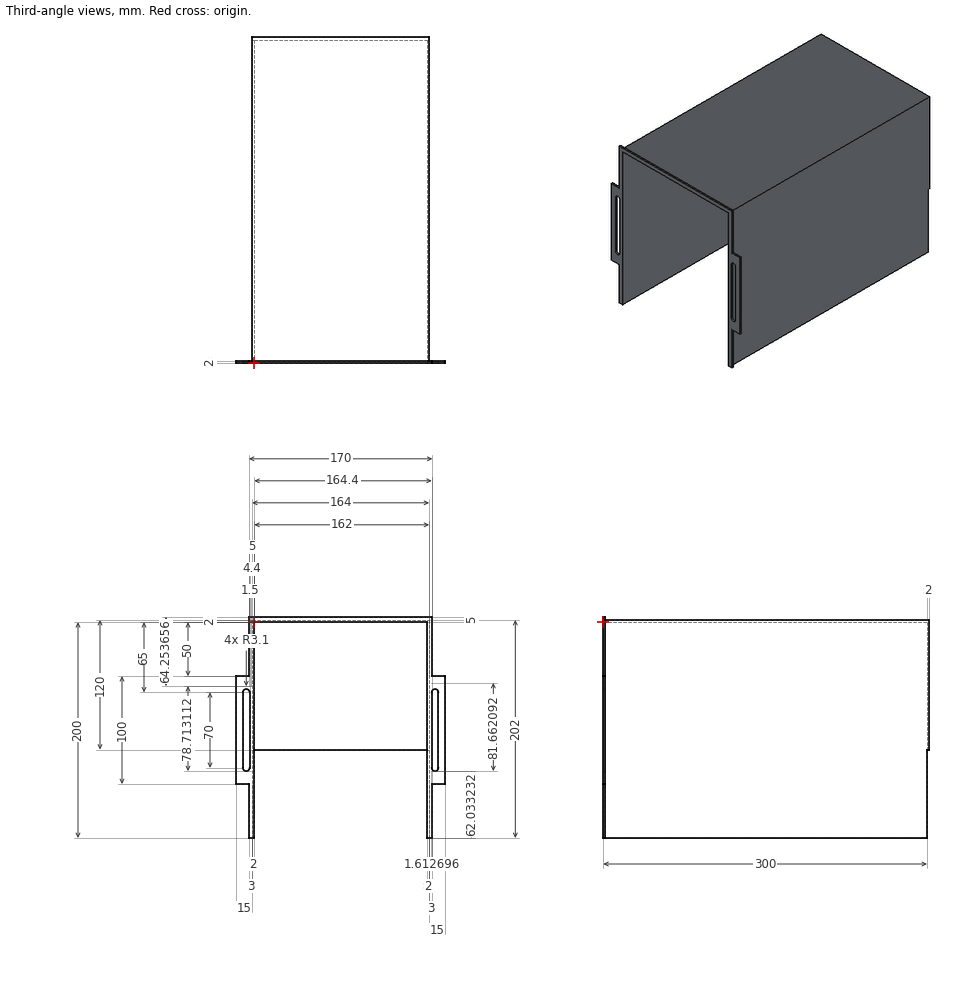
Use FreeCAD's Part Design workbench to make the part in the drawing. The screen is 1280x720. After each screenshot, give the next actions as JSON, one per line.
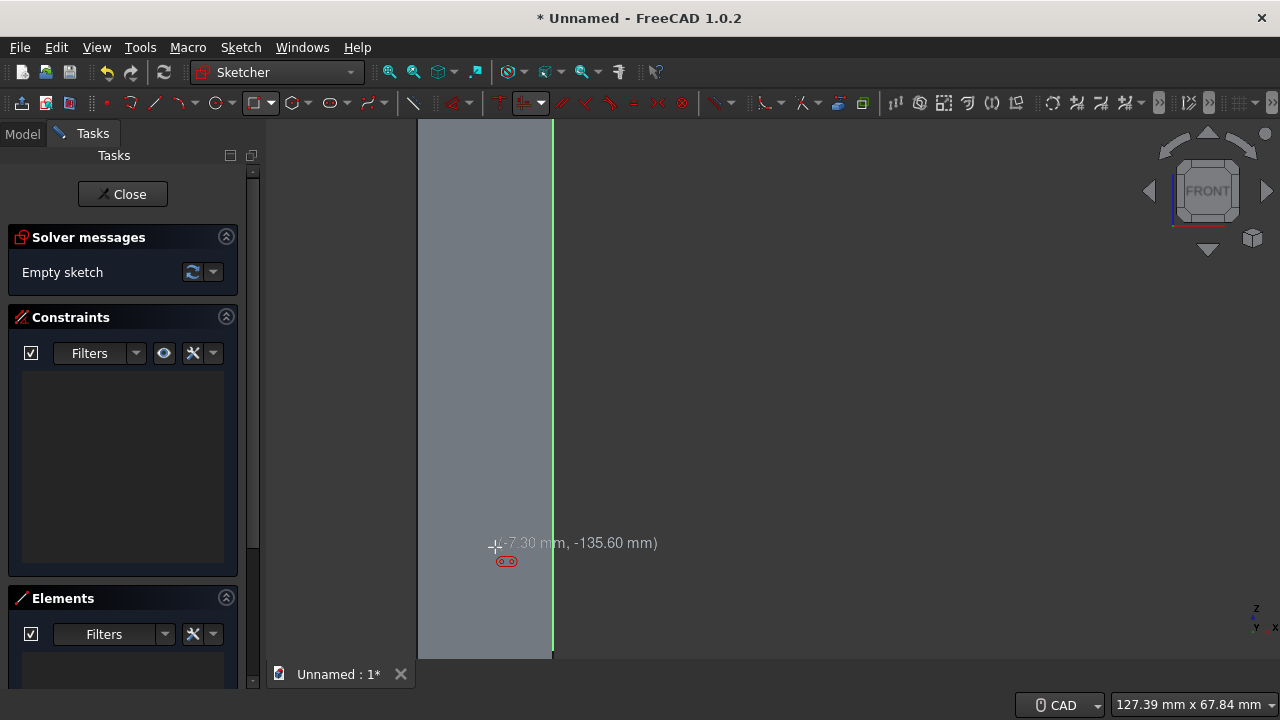
{"action": "left_click", "coordinate": [493, 544]}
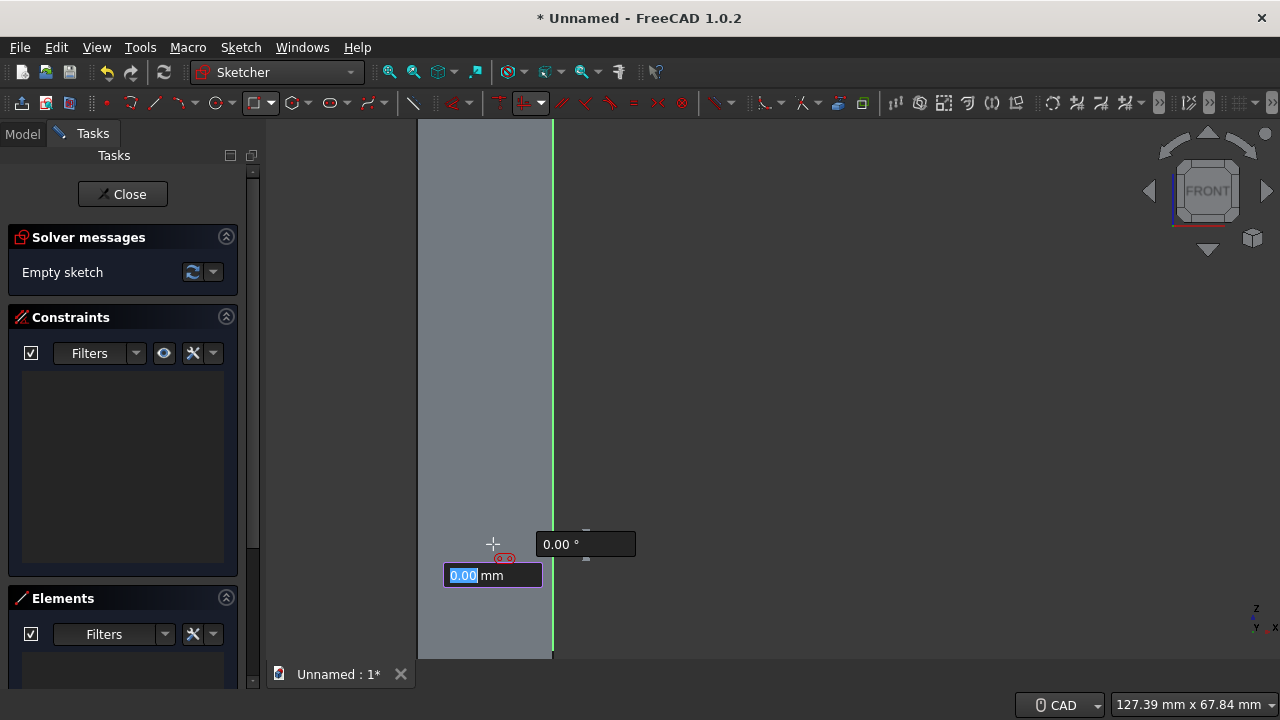
{"action": "scroll", "coordinate": [496, 549], "scroll_direction": "down", "scroll_amount": 6}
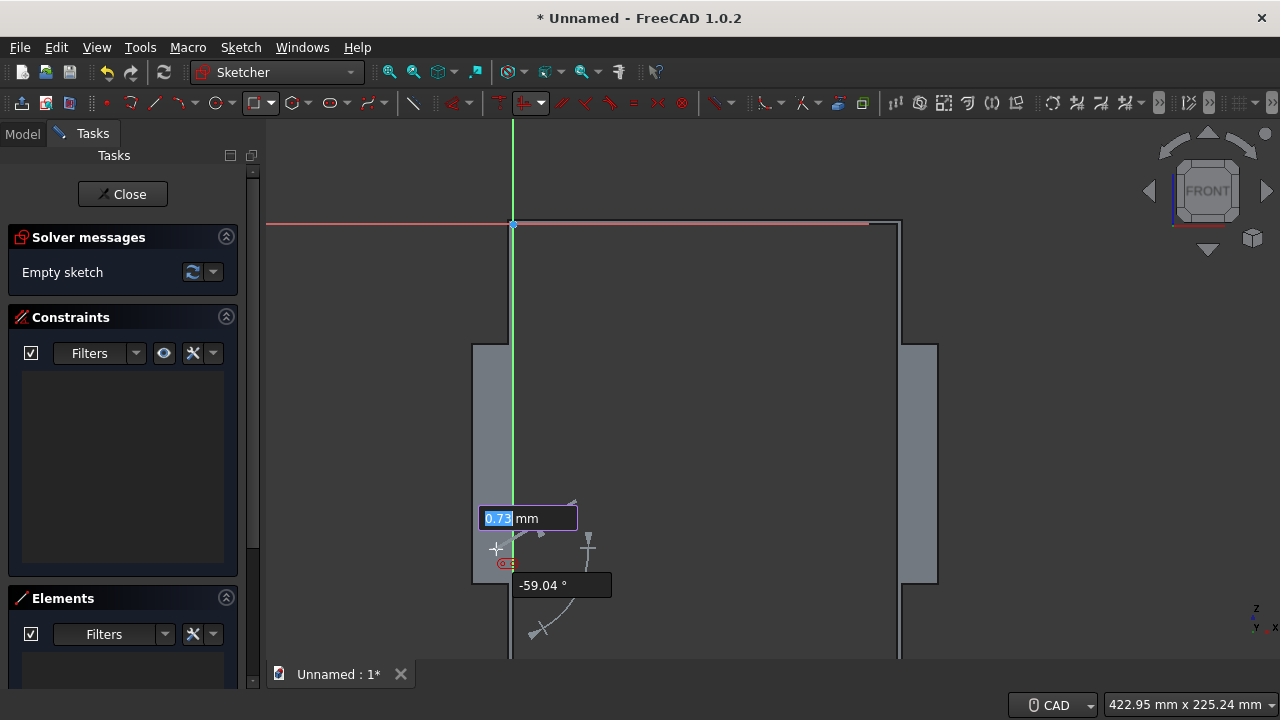
{"action": "left_click", "coordinate": [495, 380]}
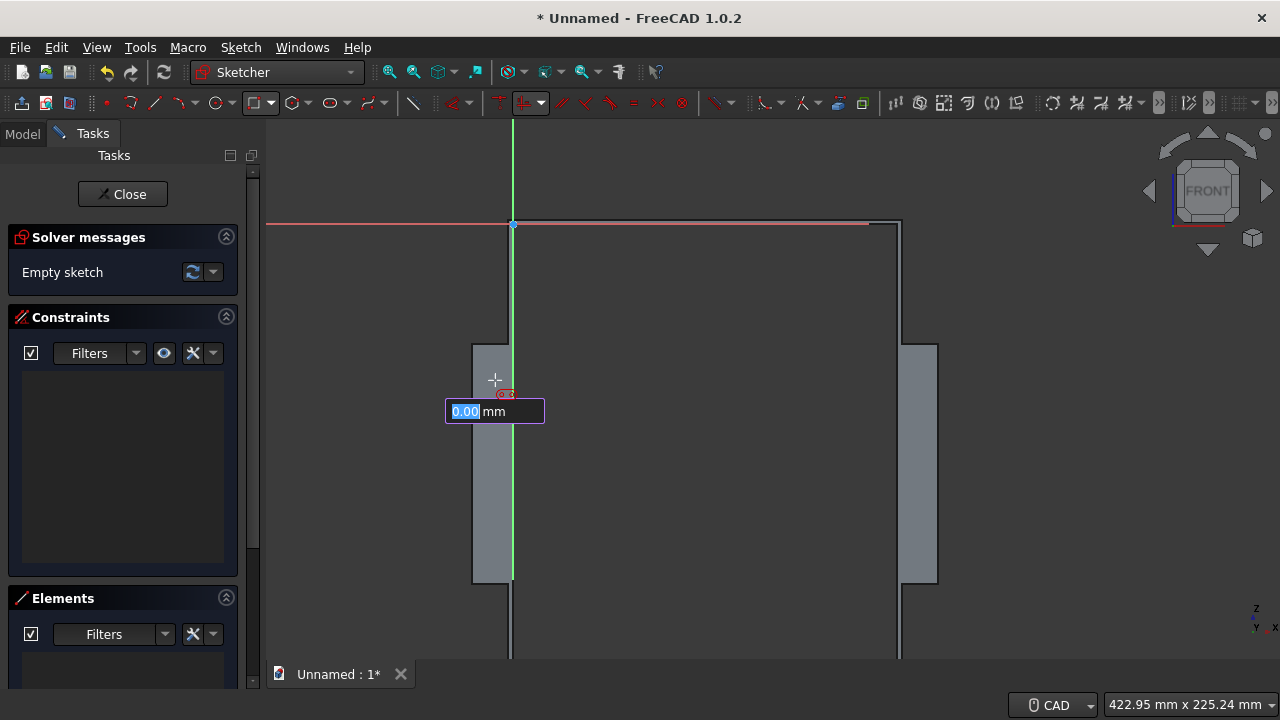
{"action": "scroll", "coordinate": [488, 464], "scroll_direction": "up", "scroll_amount": 4}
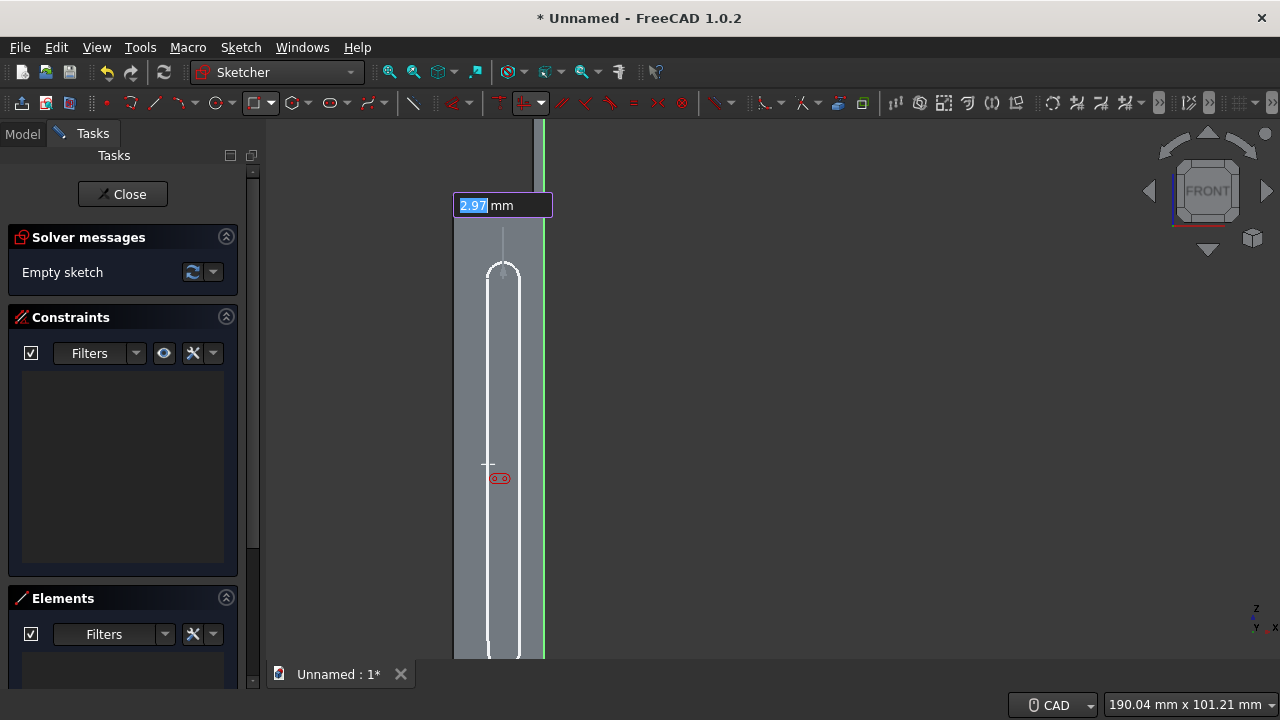
{"action": "left_click", "coordinate": [487, 463]}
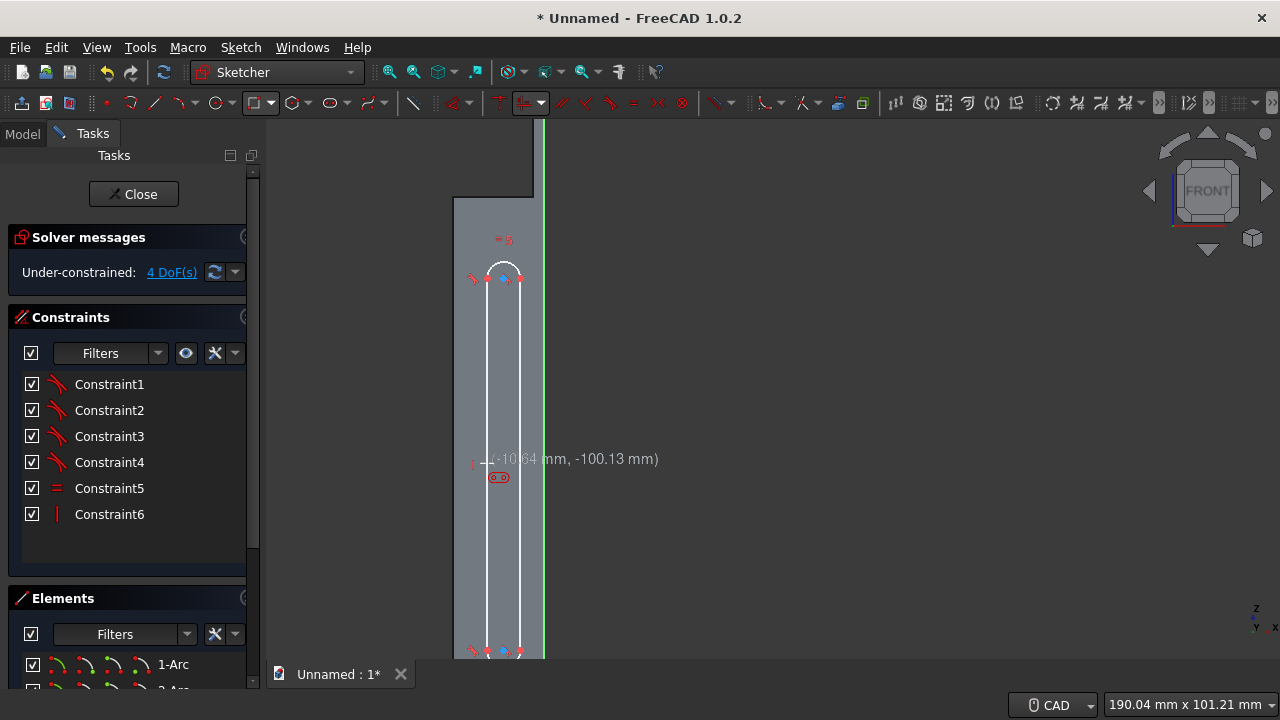
{"action": "scroll", "coordinate": [487, 463], "scroll_direction": "down", "scroll_amount": 4}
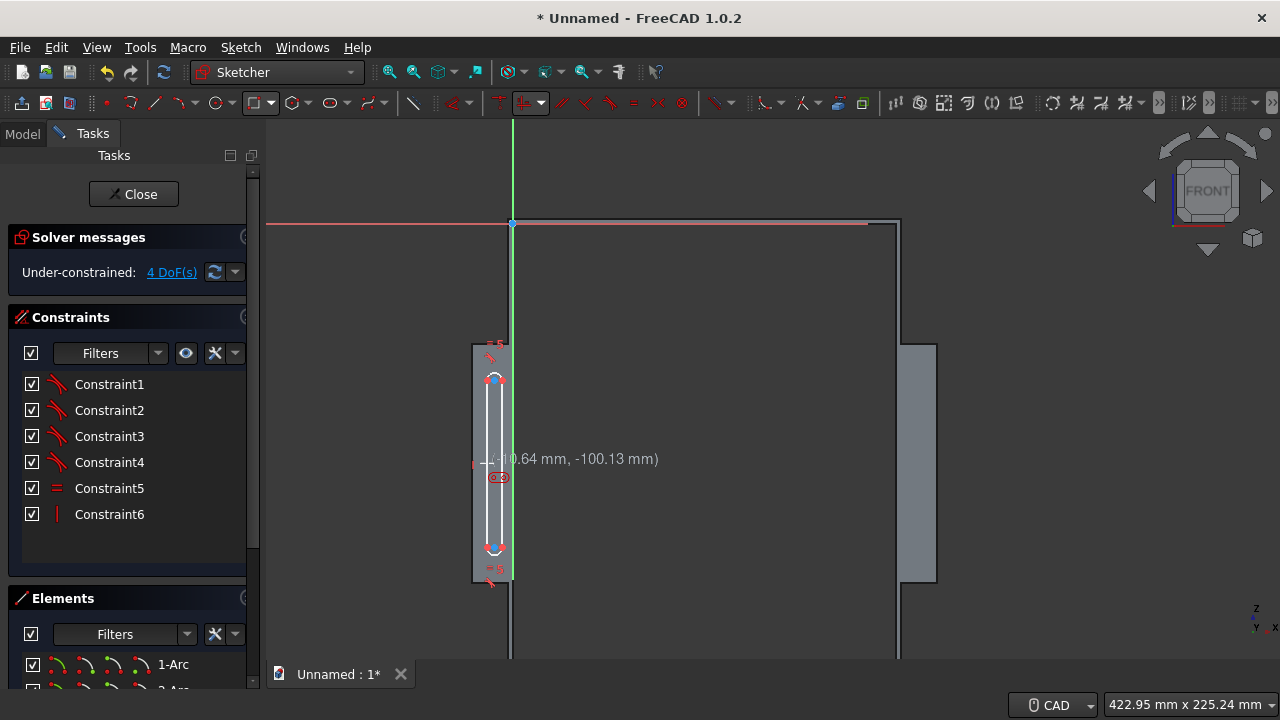
{"action": "scroll", "coordinate": [914, 547], "scroll_direction": "up", "scroll_amount": 6}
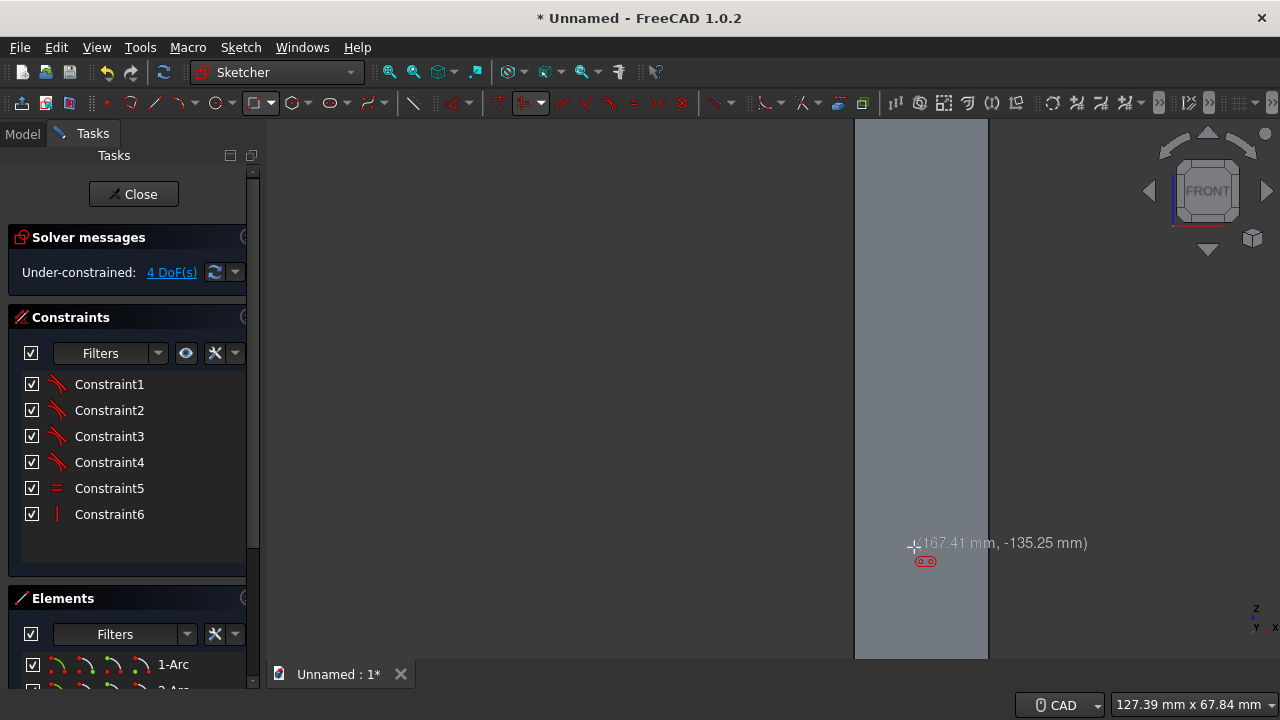
{"action": "left_click", "coordinate": [913, 546]}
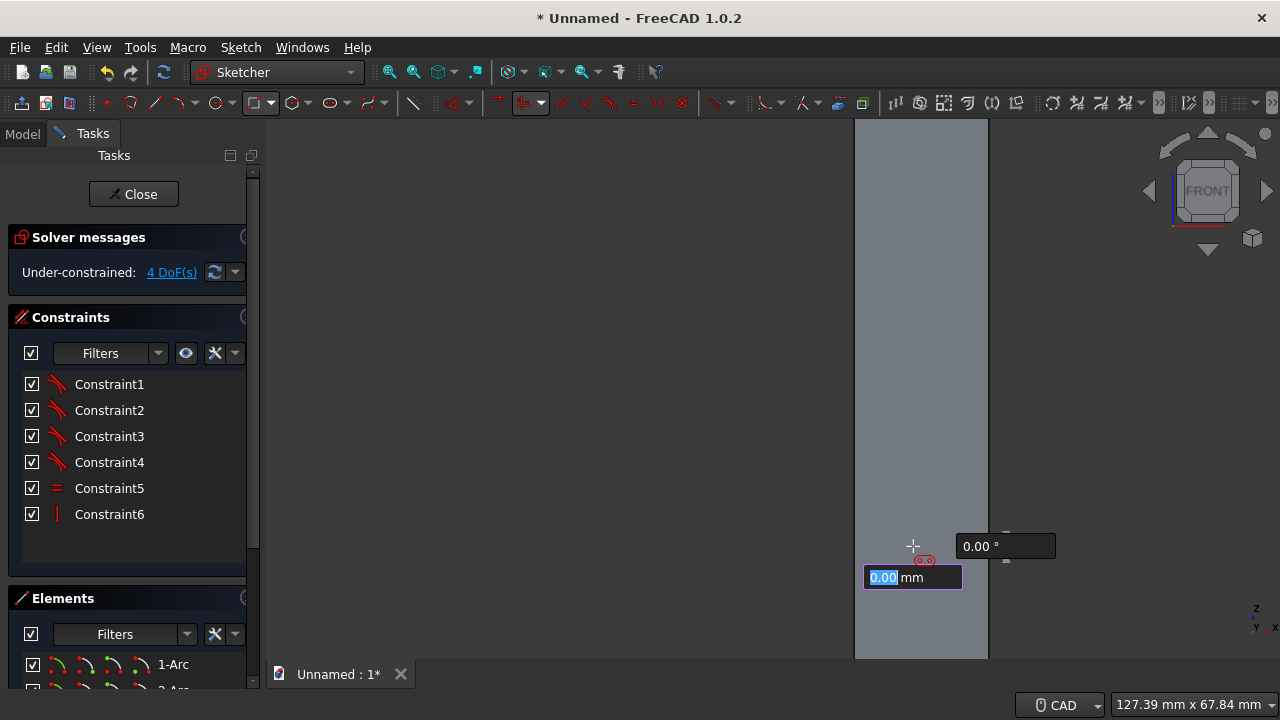
{"action": "scroll", "coordinate": [915, 547], "scroll_direction": "down", "scroll_amount": 6}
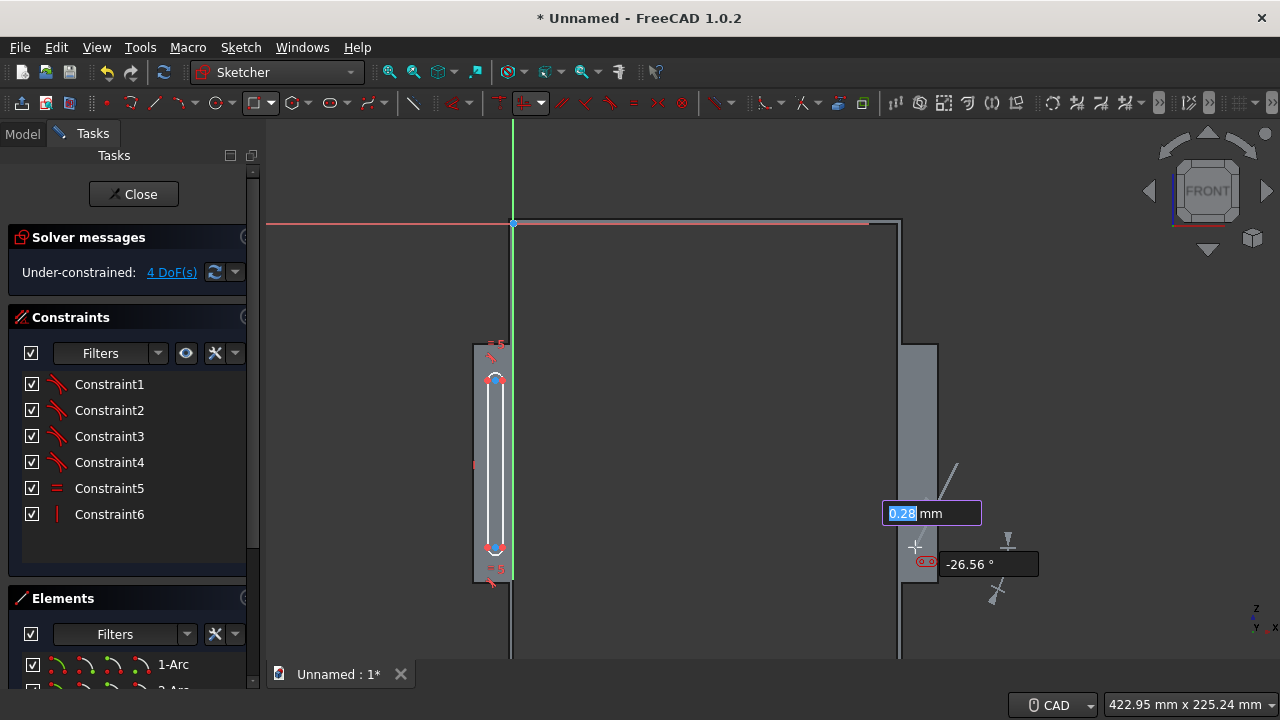
{"action": "left_click", "coordinate": [915, 380]}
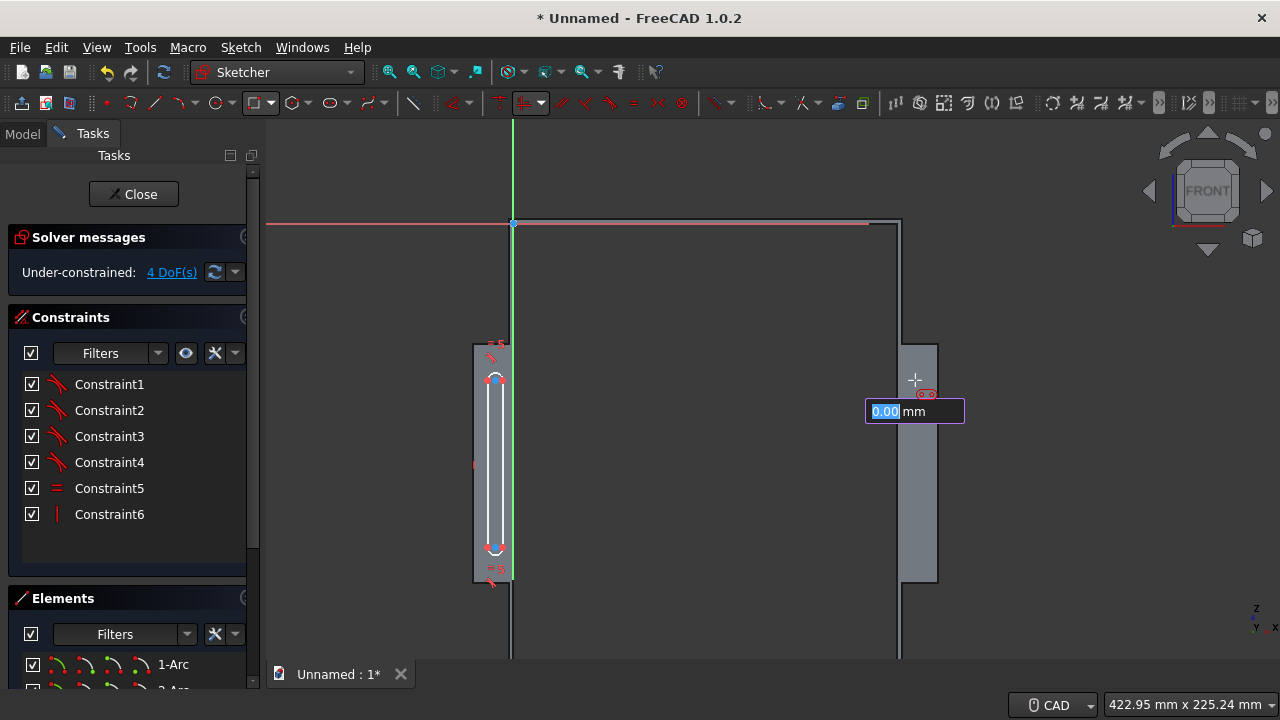
{"action": "scroll", "coordinate": [922, 463], "scroll_direction": "up", "scroll_amount": 4}